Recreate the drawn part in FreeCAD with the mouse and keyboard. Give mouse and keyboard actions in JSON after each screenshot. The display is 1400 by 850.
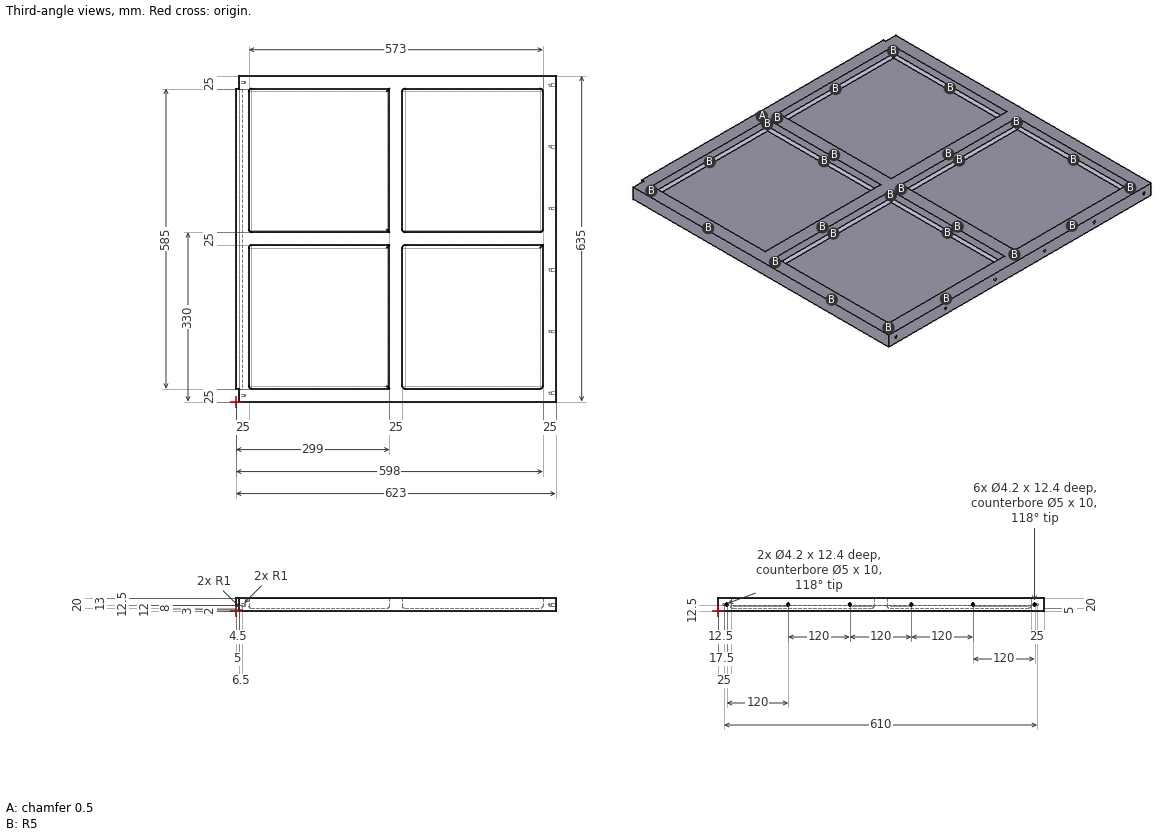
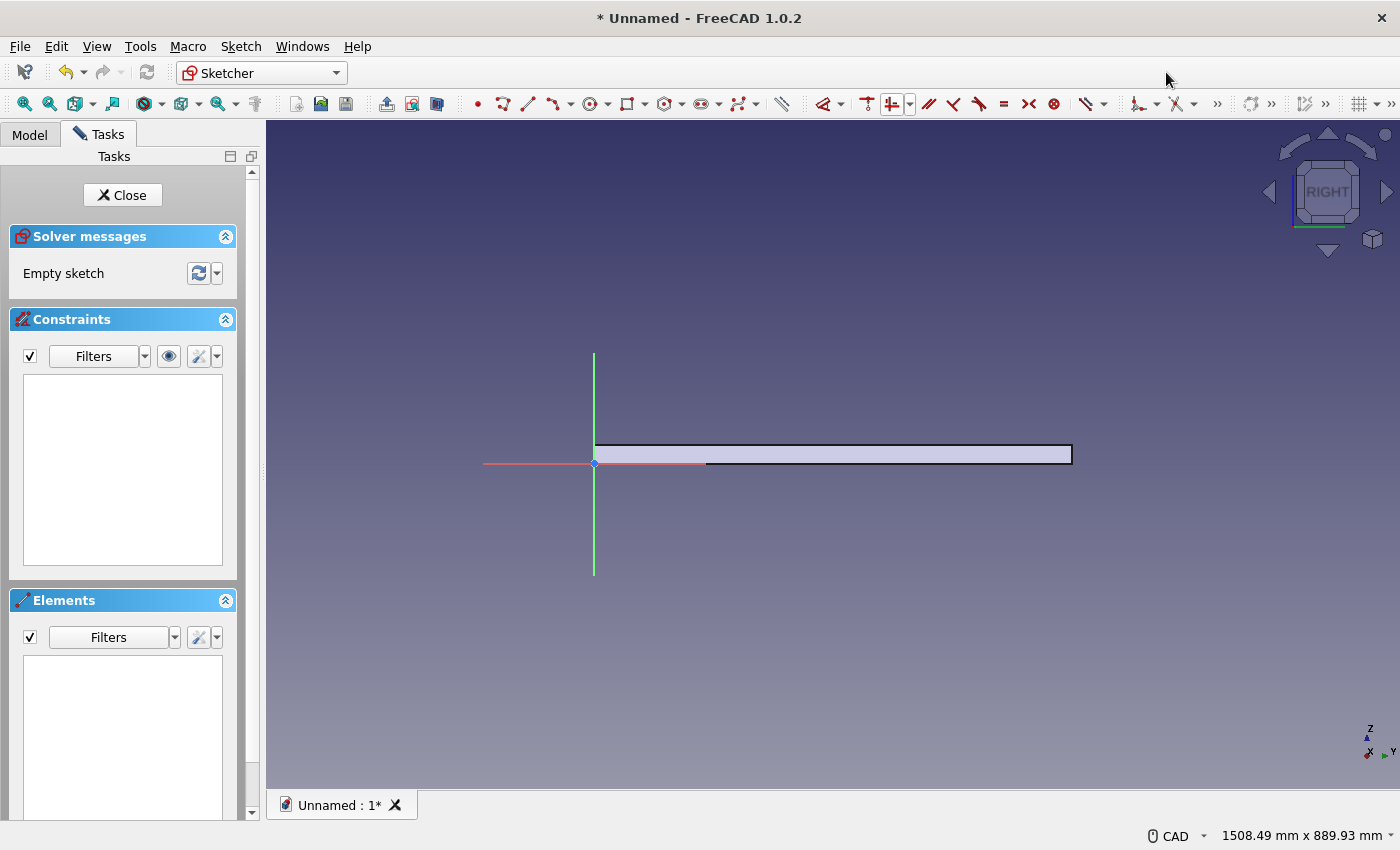
{"action": "scroll", "coordinate": [955, 466], "scroll_direction": "up", "scroll_amount": 2}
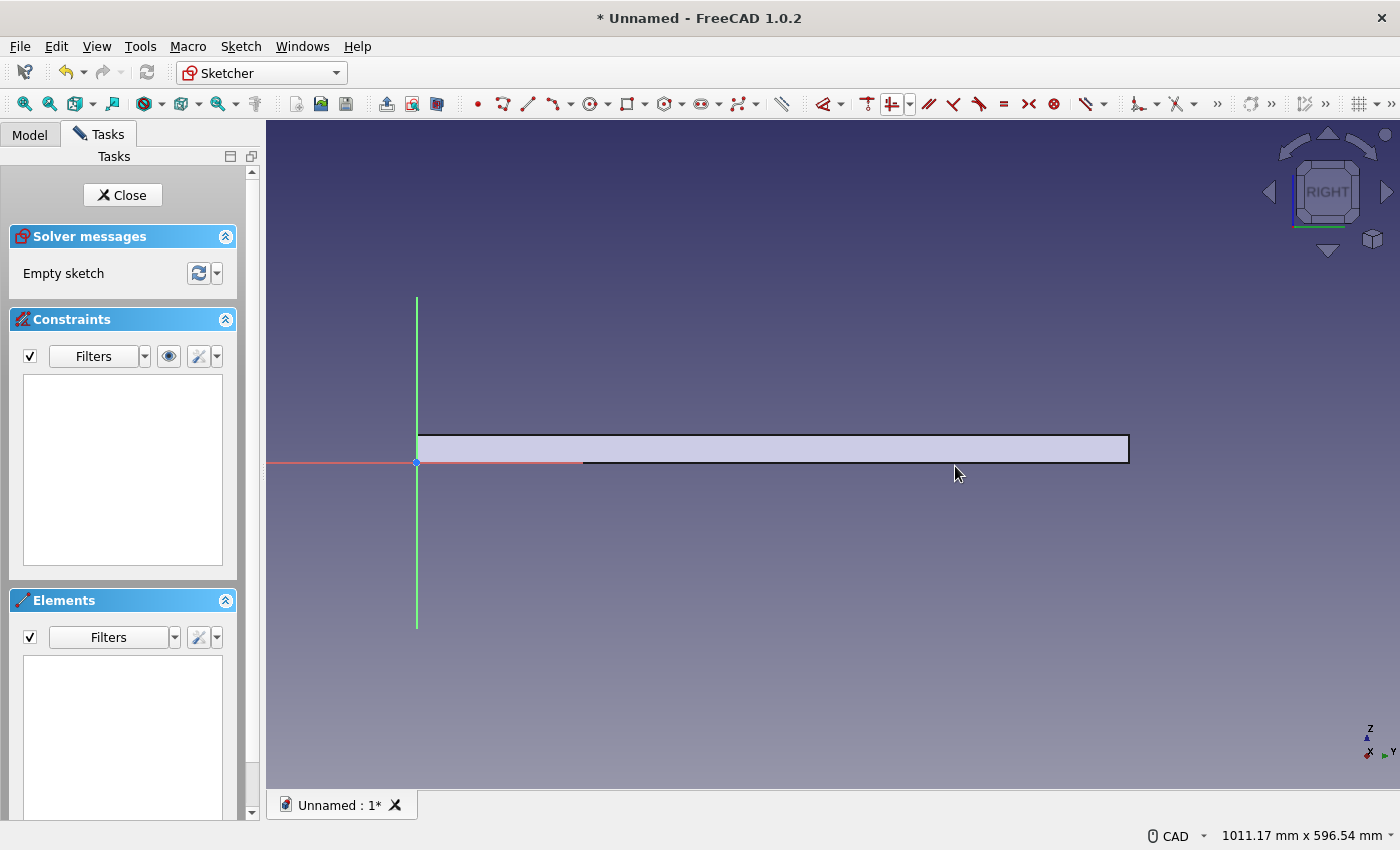
{"action": "left_click", "coordinate": [590, 104]}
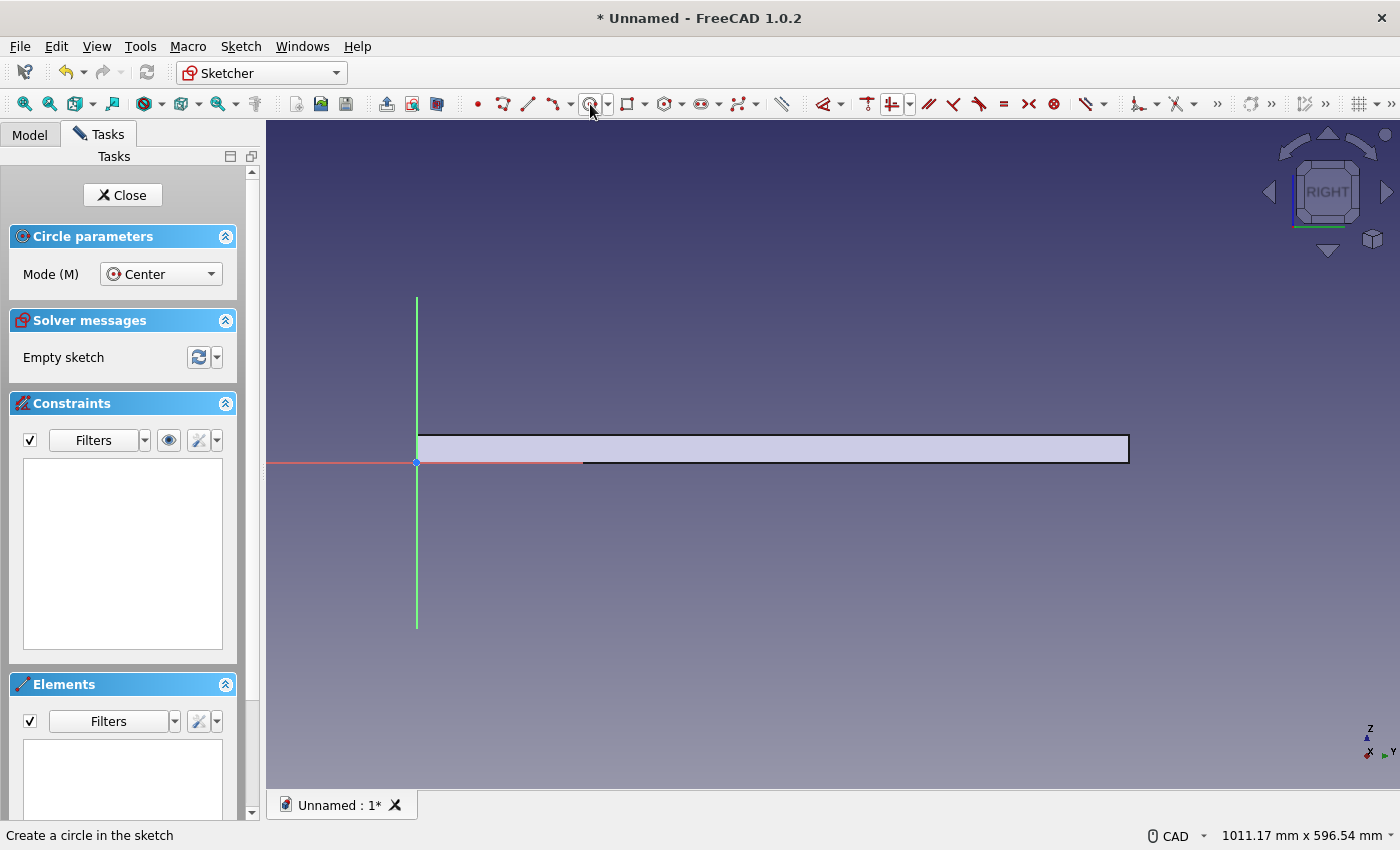
{"action": "scroll", "coordinate": [1109, 449], "scroll_direction": "up", "scroll_amount": 12}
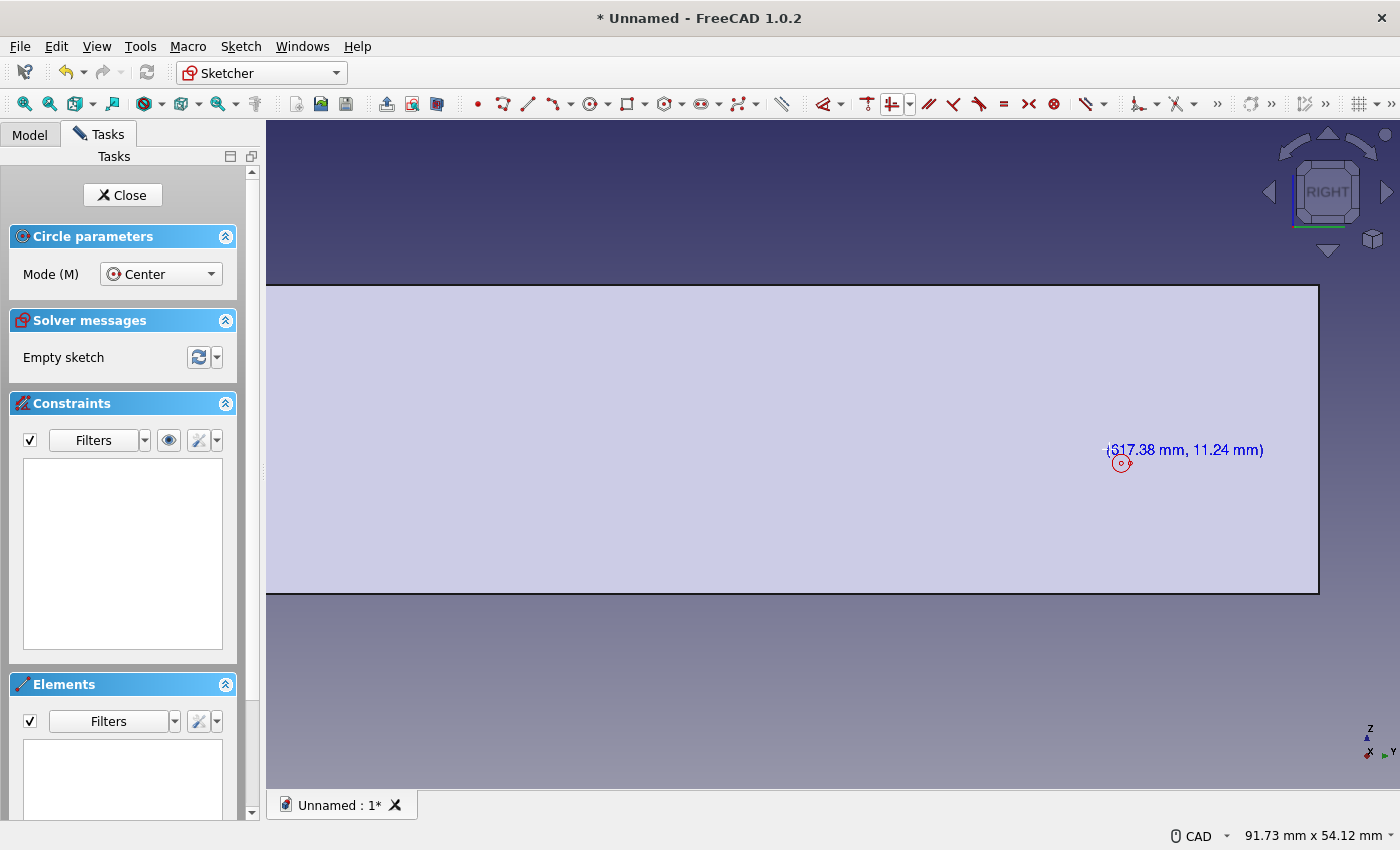
{"action": "scroll", "coordinate": [1110, 450], "scroll_direction": "down", "scroll_amount": 12}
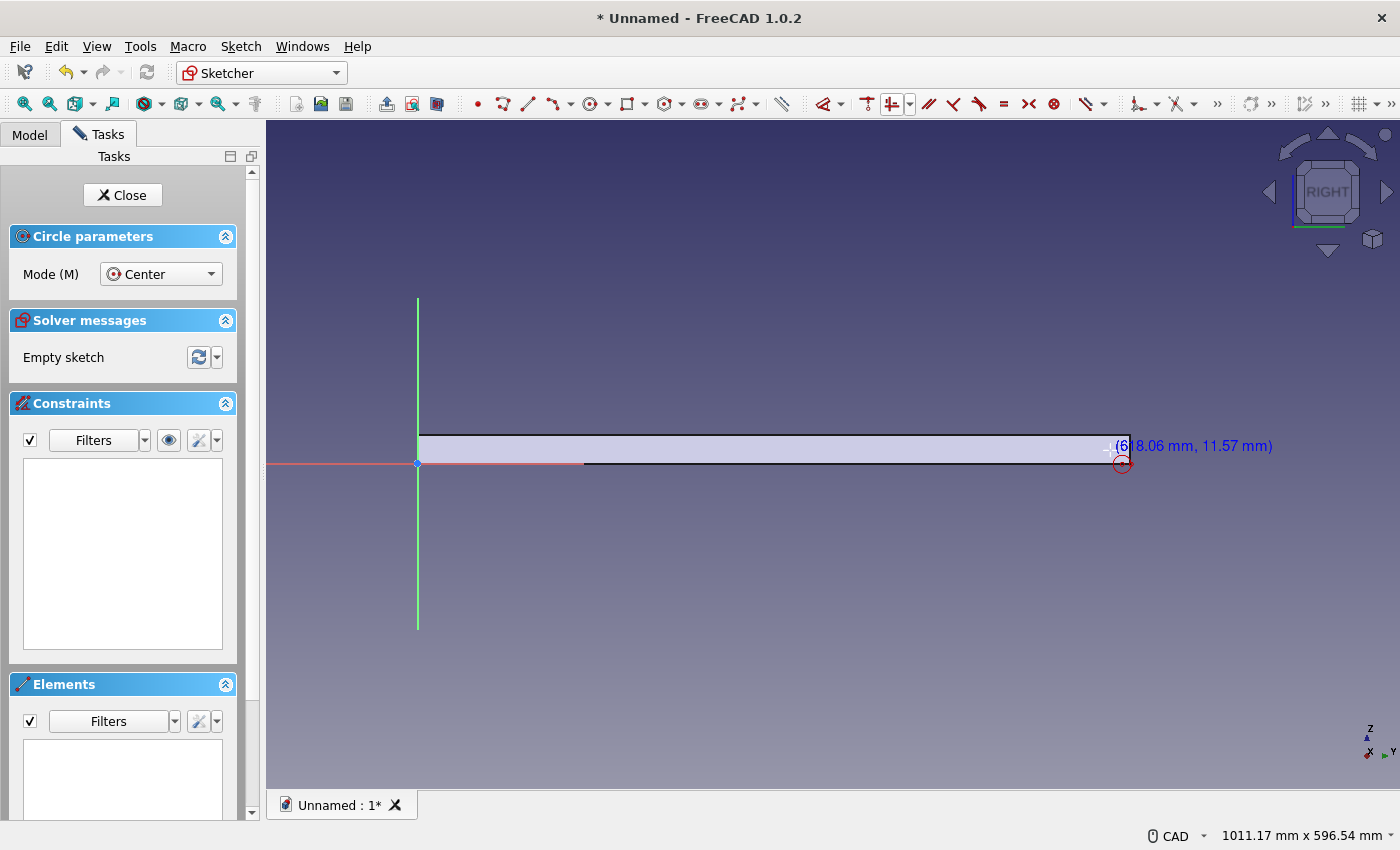
{"action": "left_click", "coordinate": [1110, 449]}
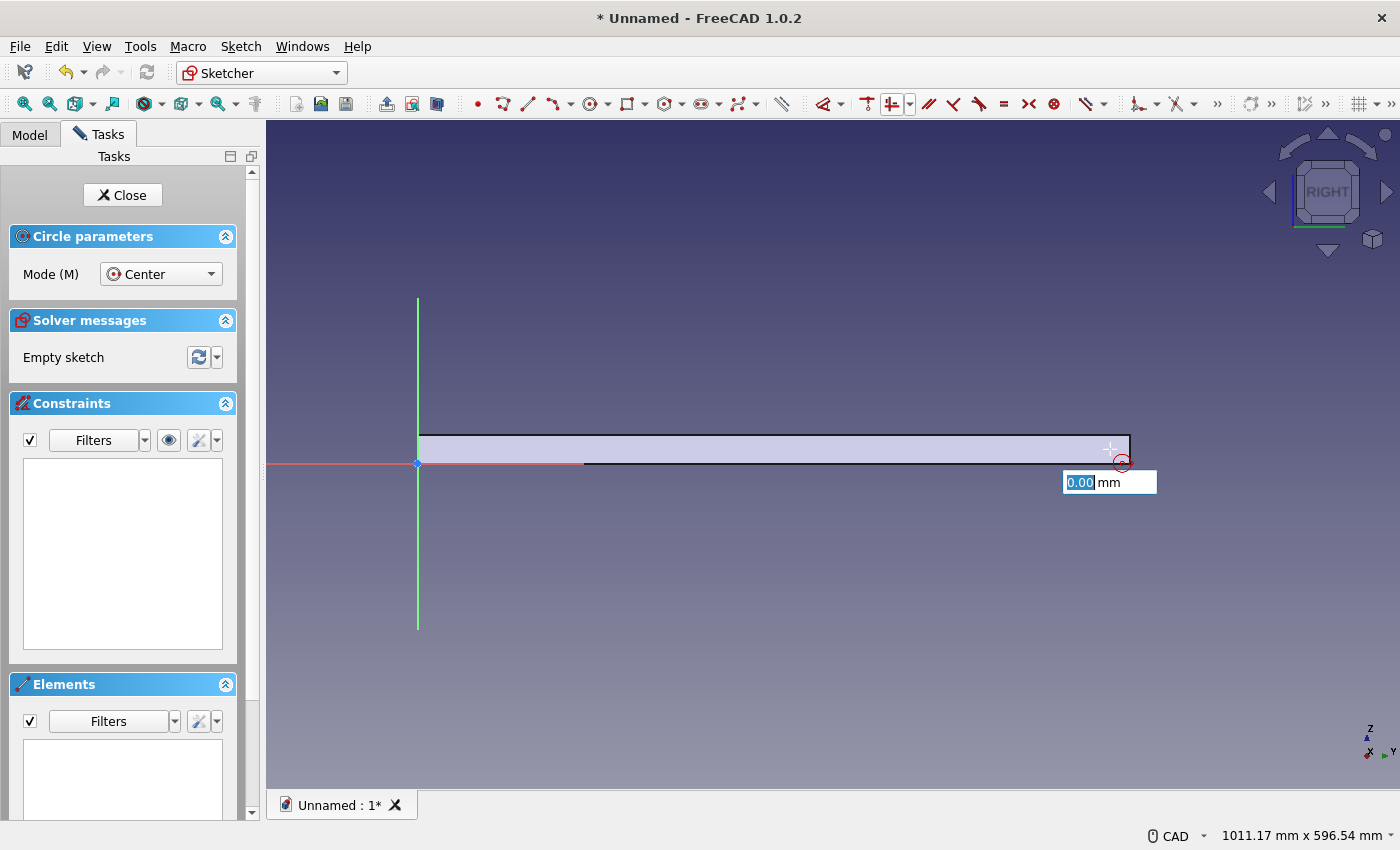
{"action": "scroll", "coordinate": [1112, 448], "scroll_direction": "up", "scroll_amount": 10}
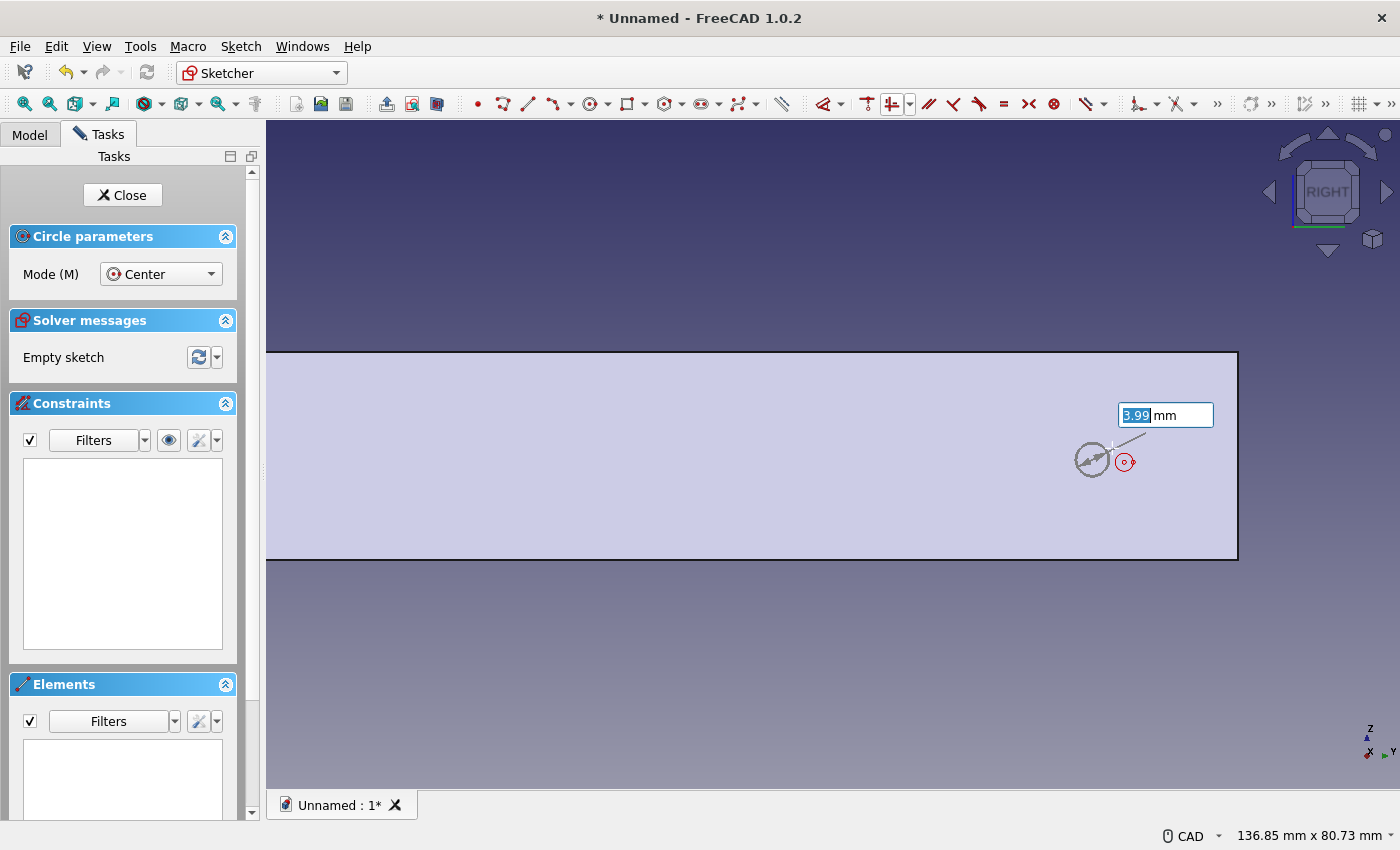
{"action": "left_click", "coordinate": [1105, 444]}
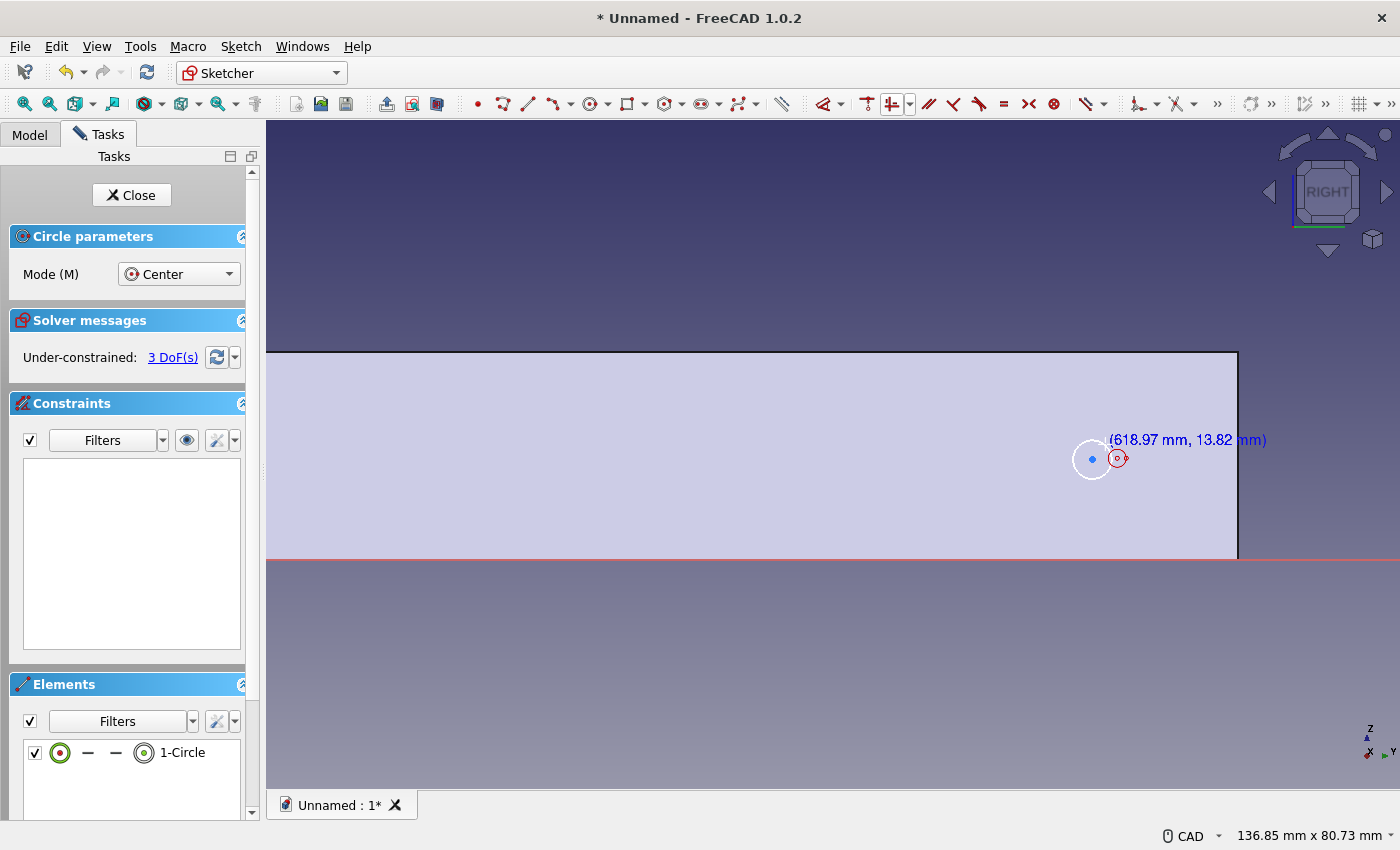
{"action": "scroll", "coordinate": [1112, 448], "scroll_direction": "down", "scroll_amount": 10}